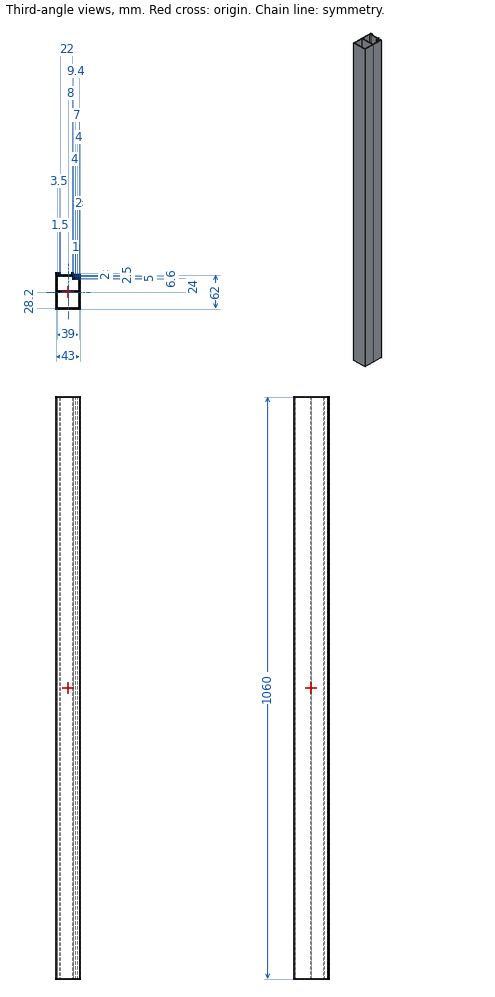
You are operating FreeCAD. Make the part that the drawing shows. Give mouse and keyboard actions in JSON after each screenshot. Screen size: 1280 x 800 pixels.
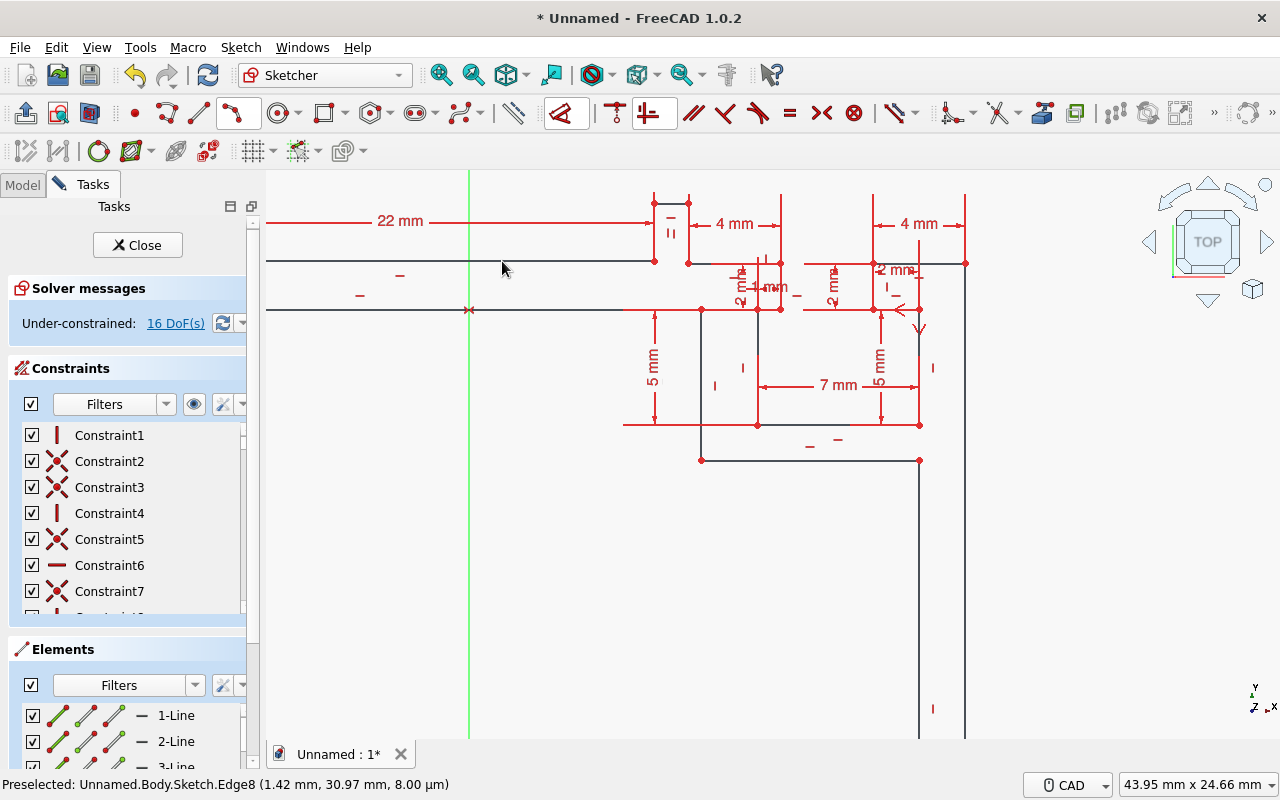
{"action": "scroll", "coordinate": [781, 293], "scroll_direction": "down", "scroll_amount": 7}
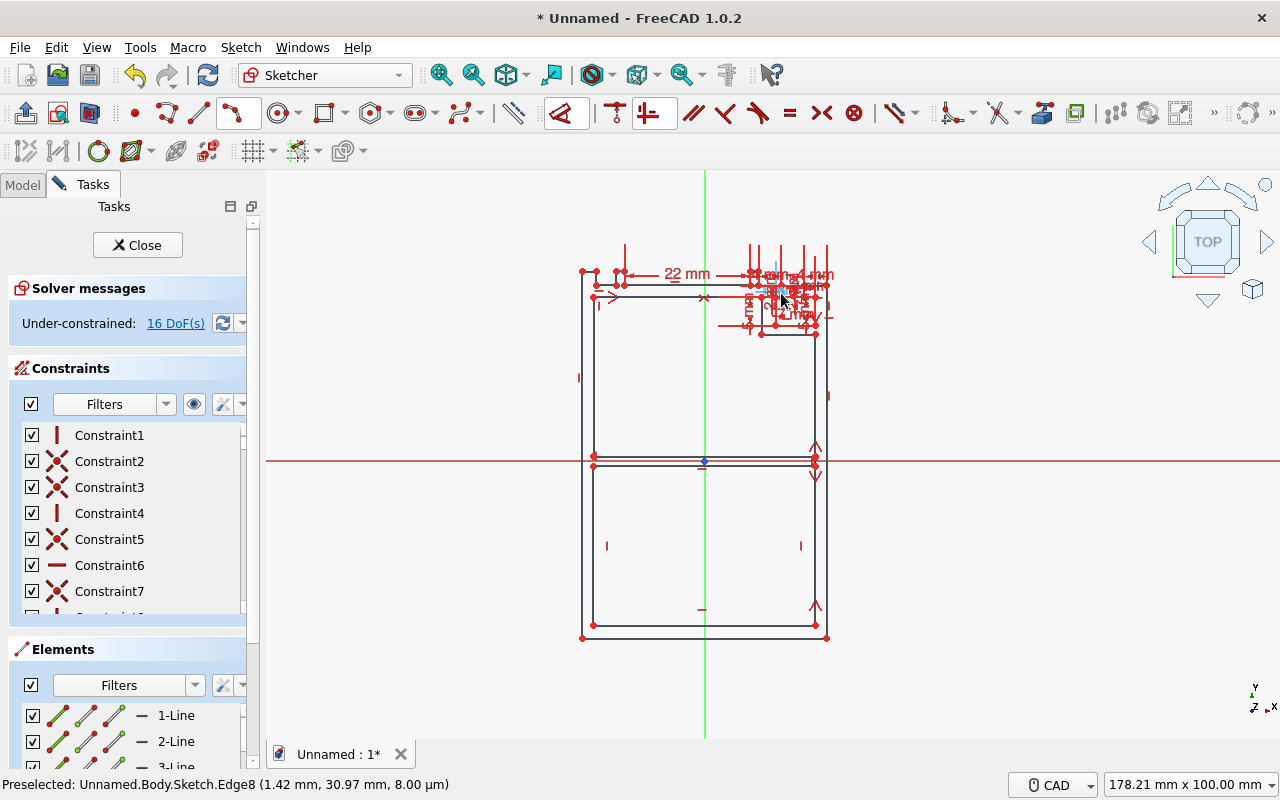
{"action": "left_click", "coordinate": [656, 639]}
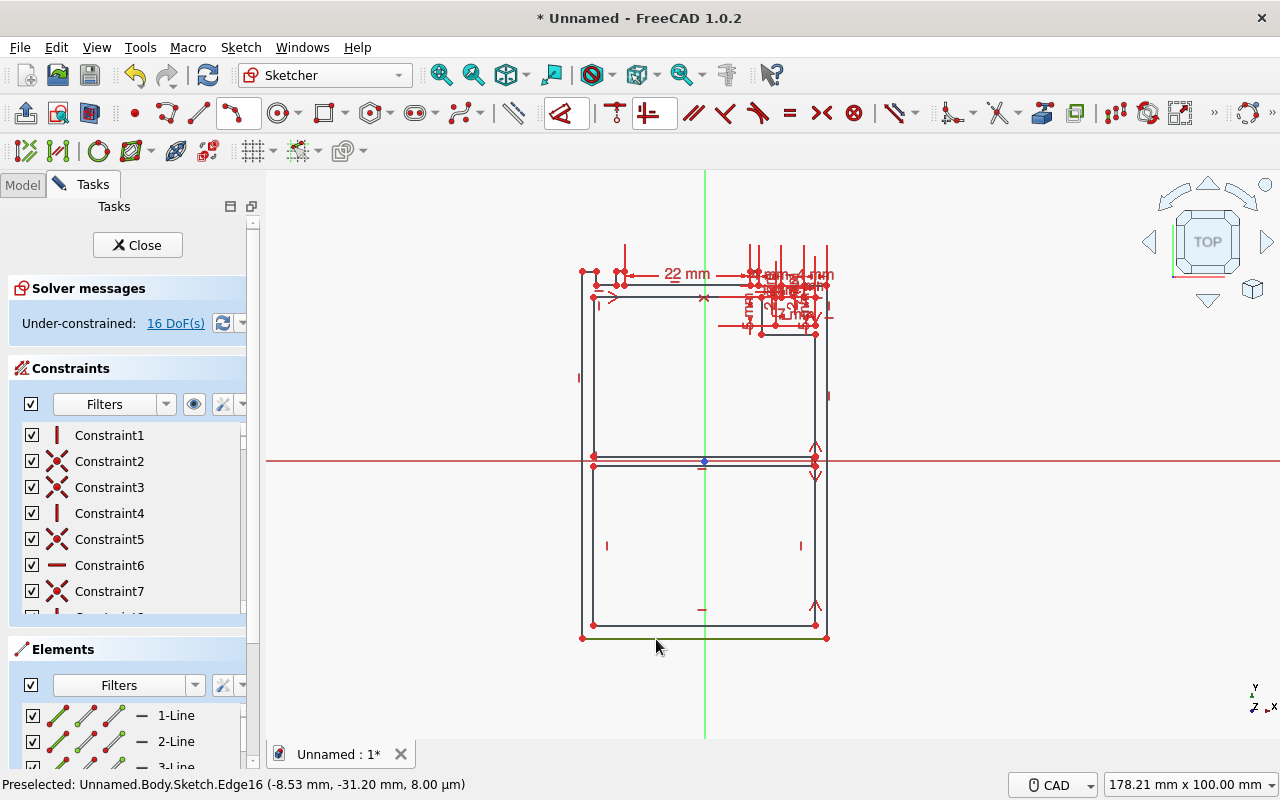
{"action": "left_click", "coordinate": [584, 114]}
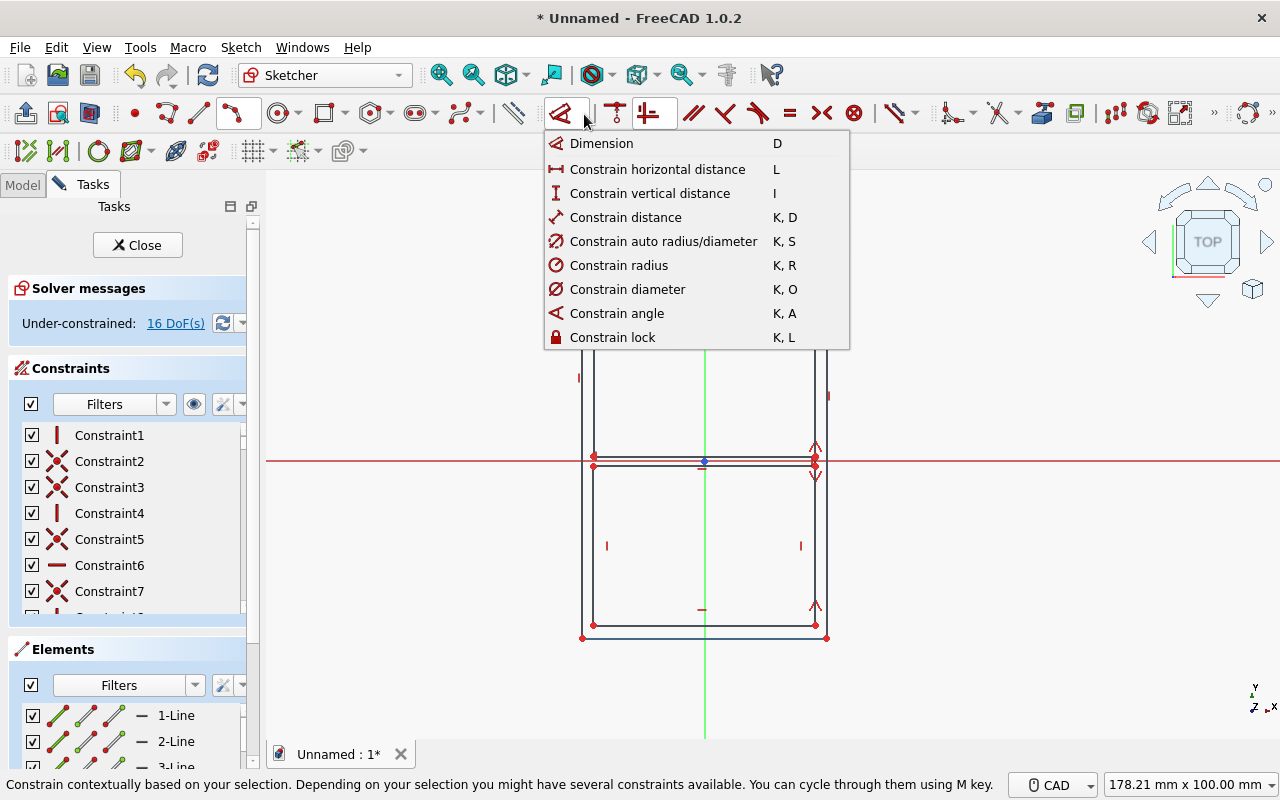
{"action": "left_click", "coordinate": [697, 169]}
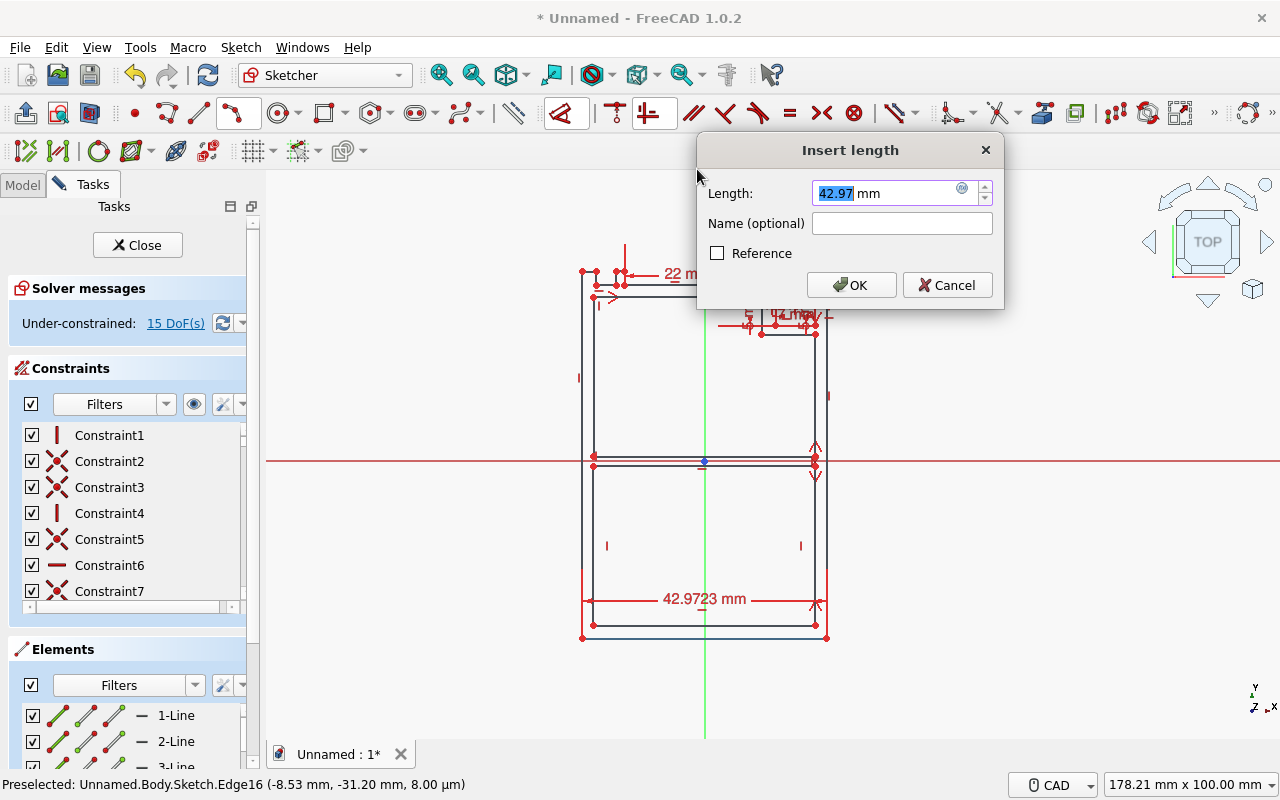
{"action": "type", "text": "43"}
{"action": "key", "text": "Return"}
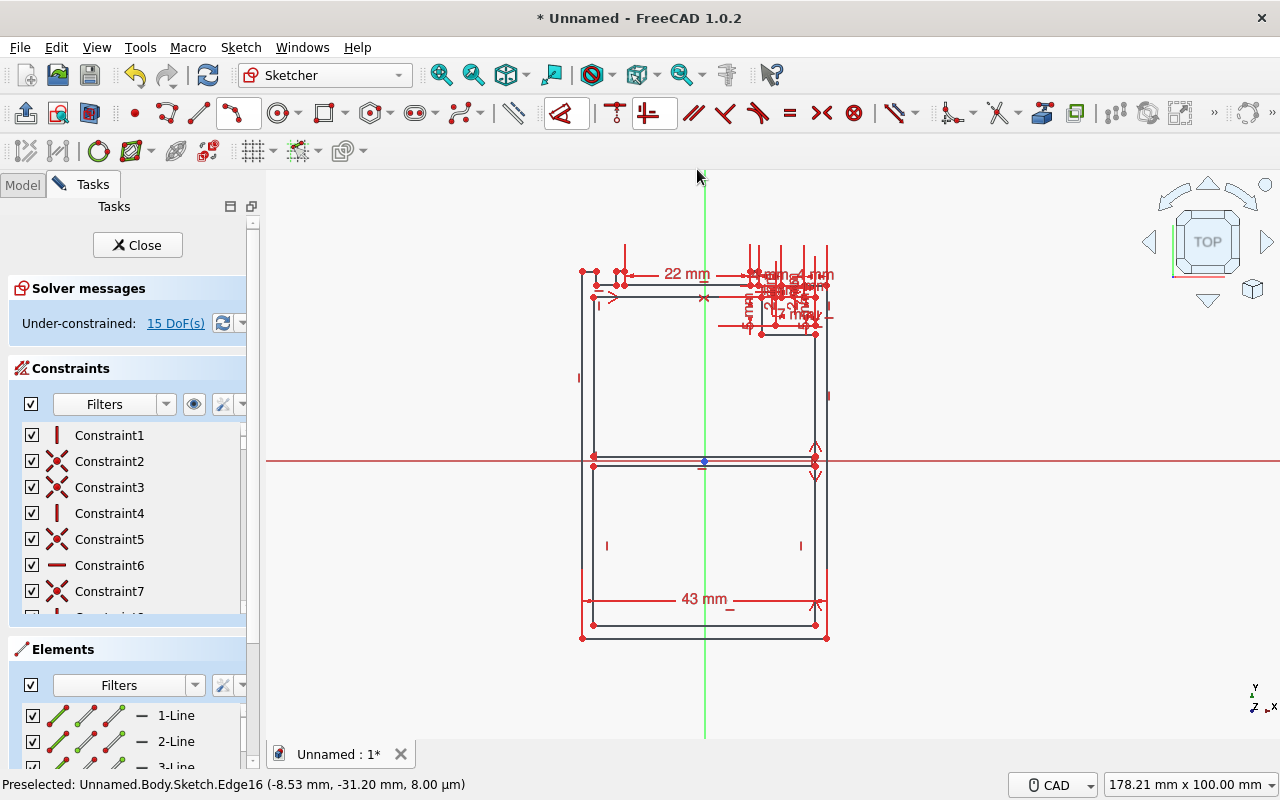
{"action": "left_click", "coordinate": [827, 533]}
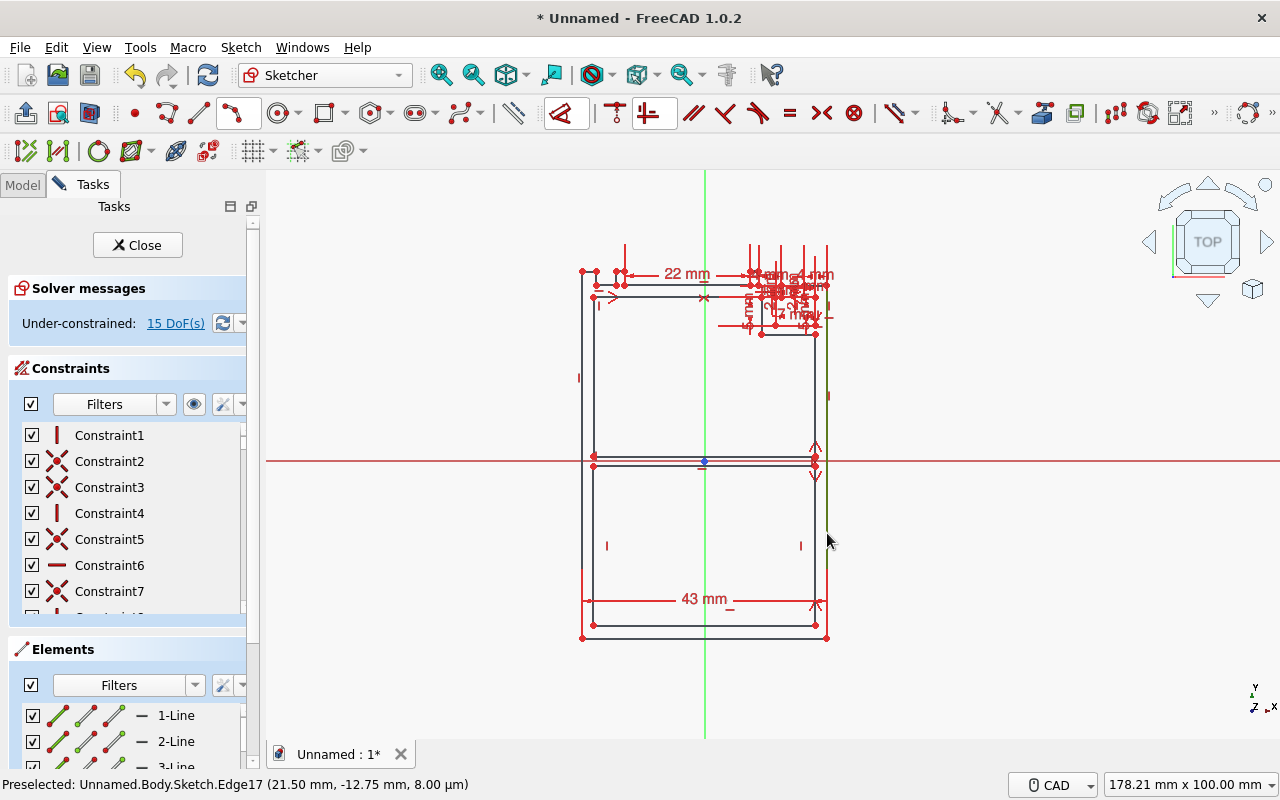
{"action": "key", "text": "i"}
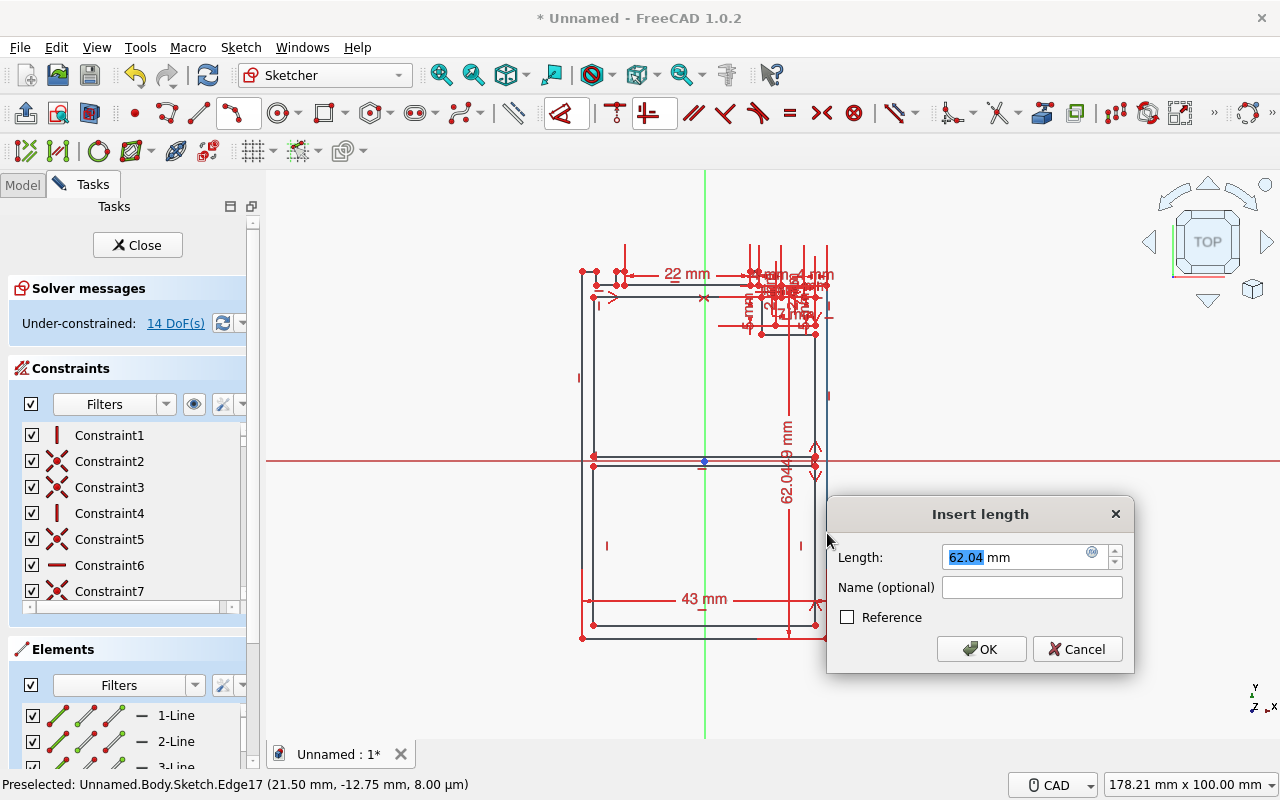
{"action": "type", "text": "62"}
{"action": "key", "text": "Return"}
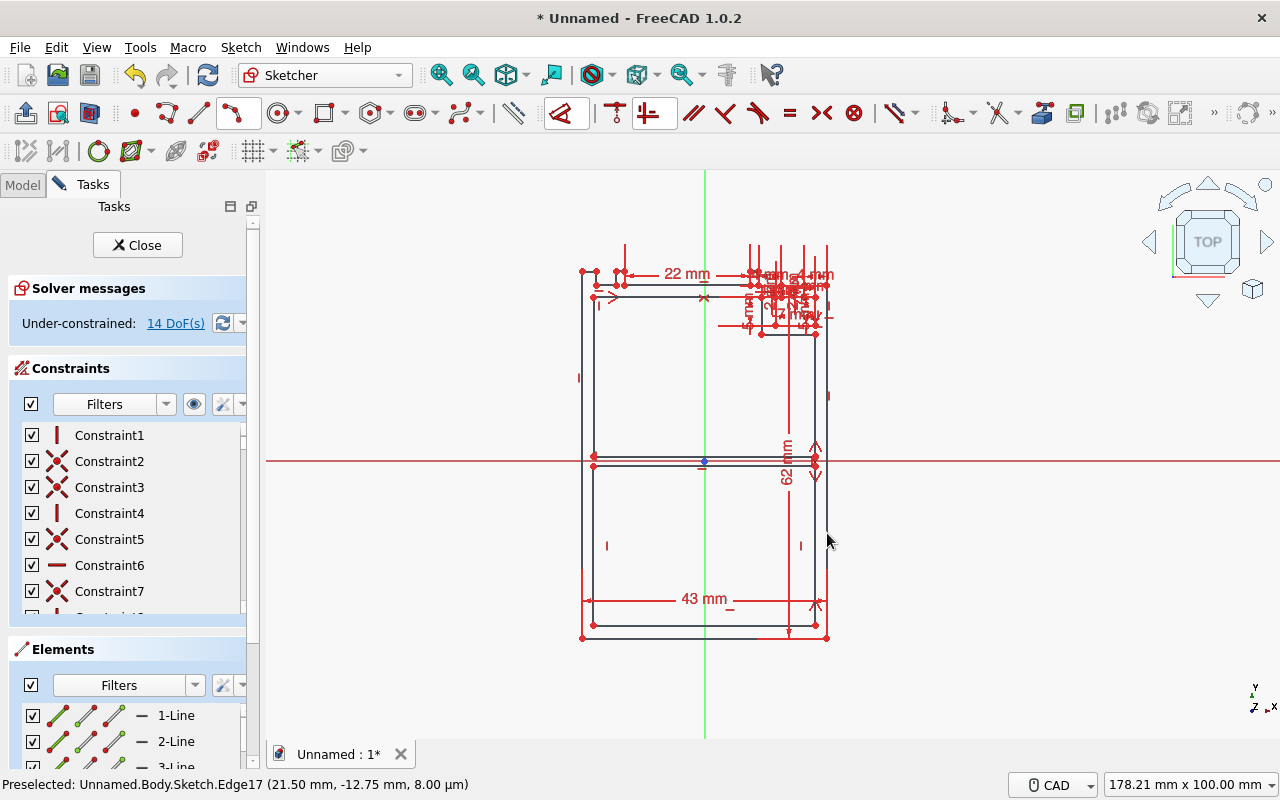
{"action": "left_click", "coordinate": [660, 626]}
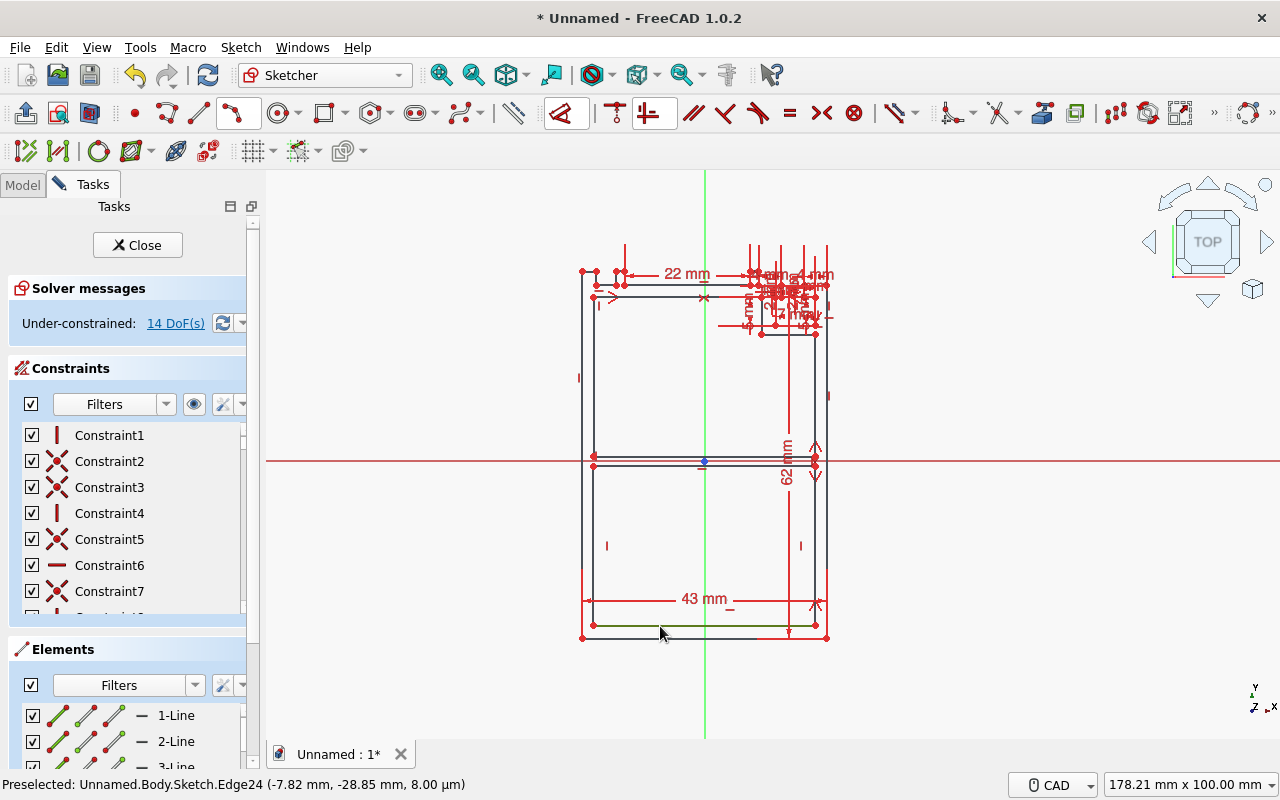
{"action": "left_click", "coordinate": [584, 114]}